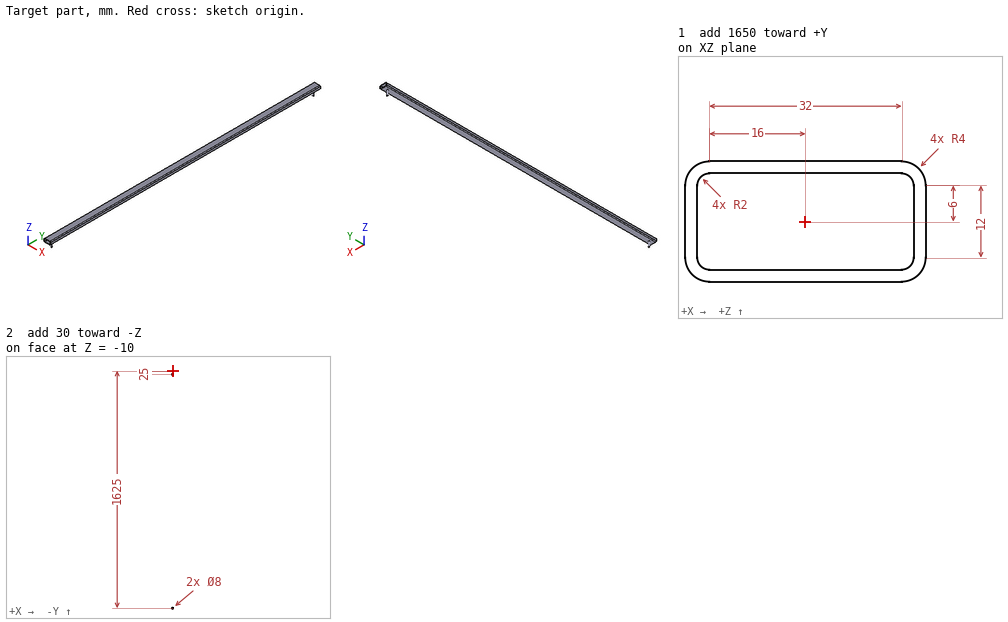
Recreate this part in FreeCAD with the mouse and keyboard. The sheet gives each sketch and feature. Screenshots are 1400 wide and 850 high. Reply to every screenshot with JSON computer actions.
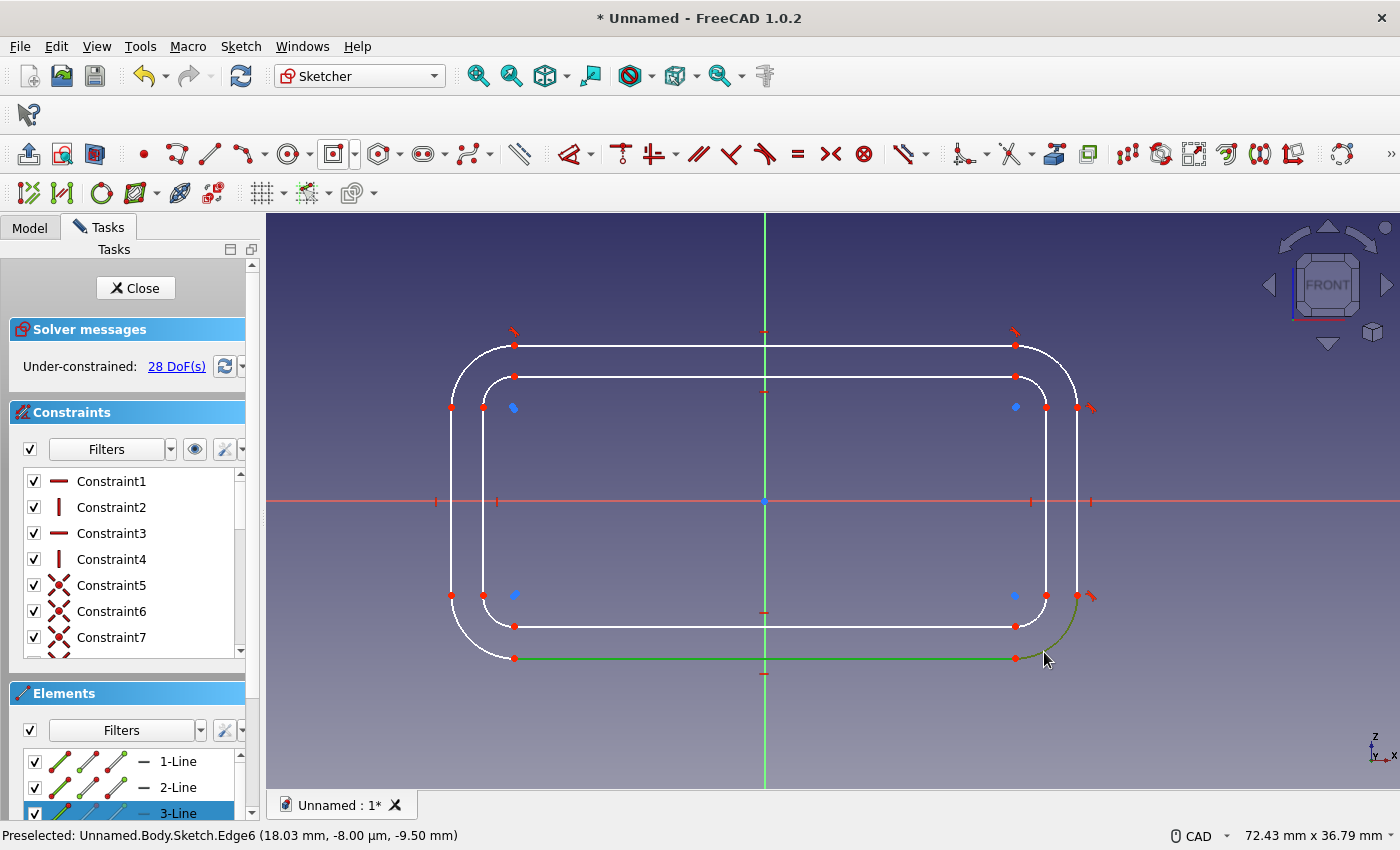
{"action": "left_click", "coordinate": [765, 154]}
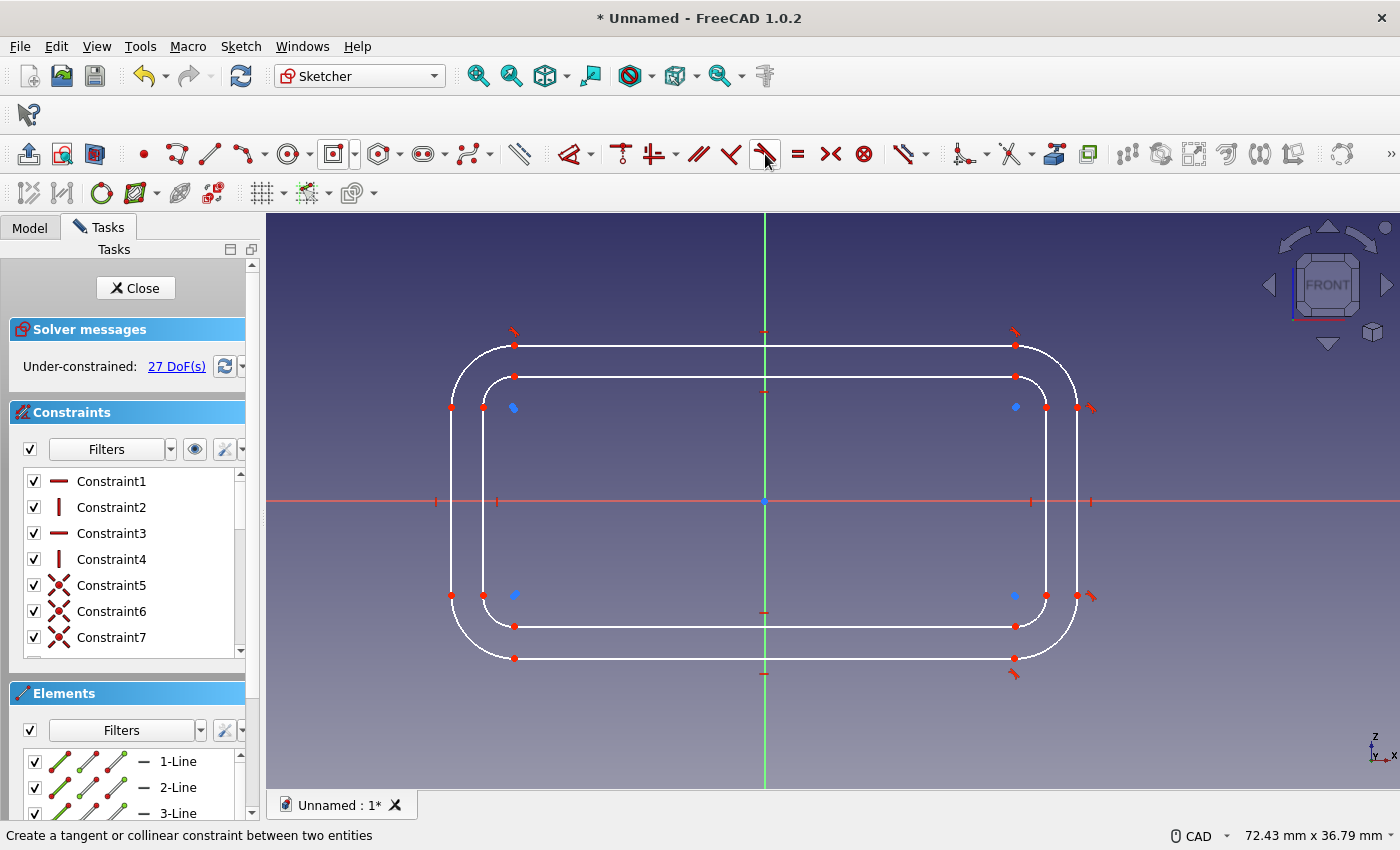
{"action": "left_click", "coordinate": [864, 659]}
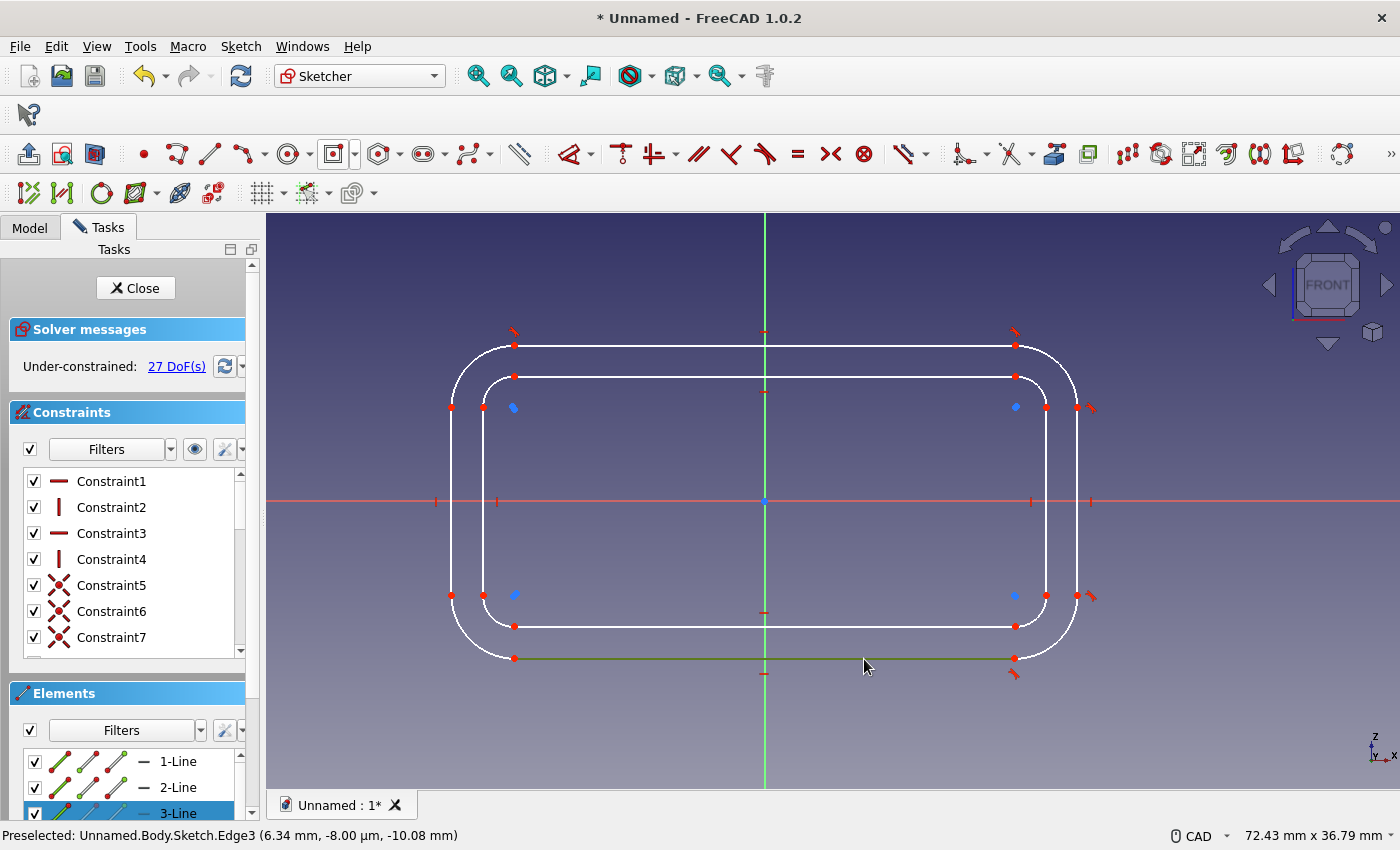
{"action": "left_click", "coordinate": [459, 624]}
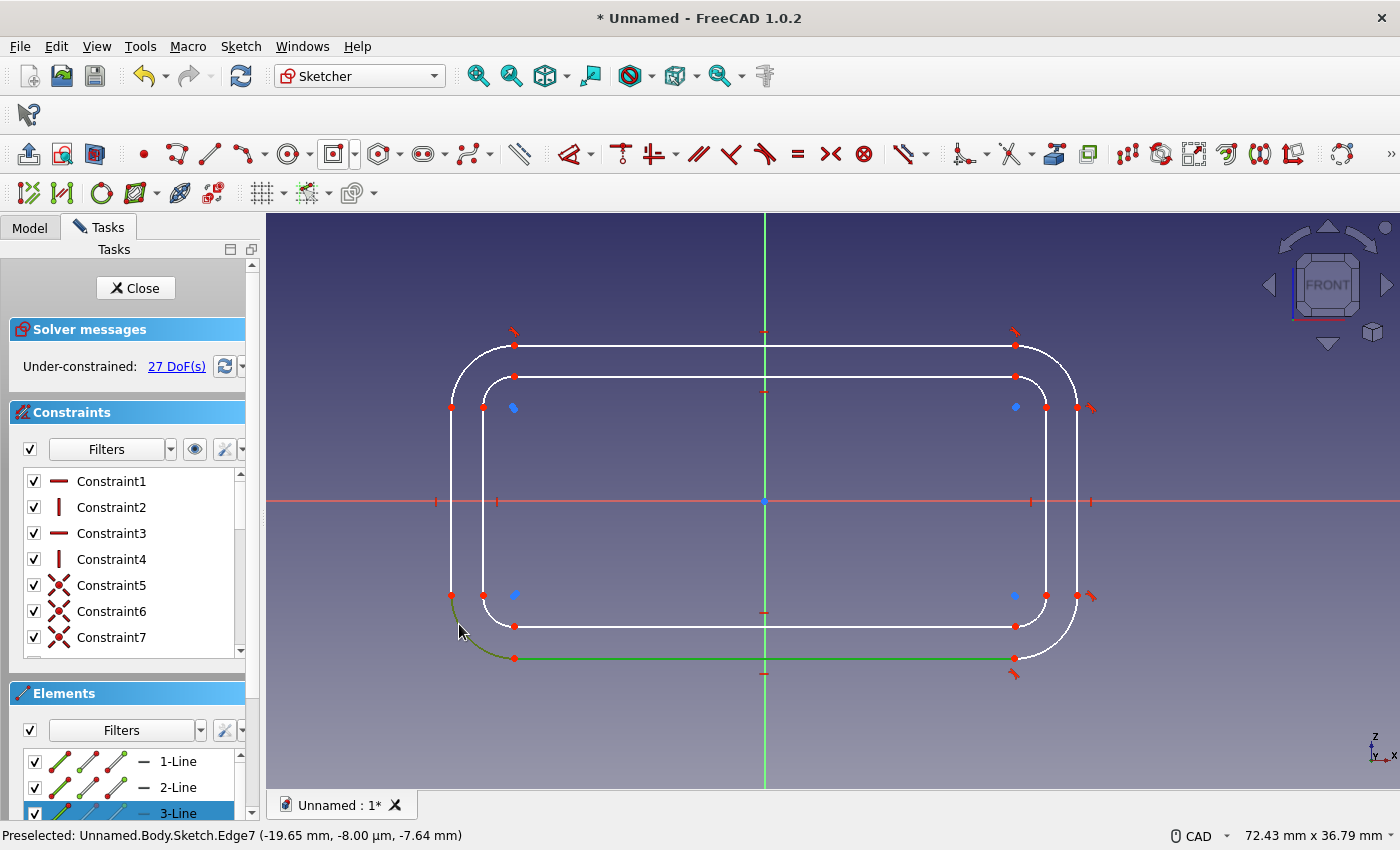
{"action": "left_click", "coordinate": [765, 154]}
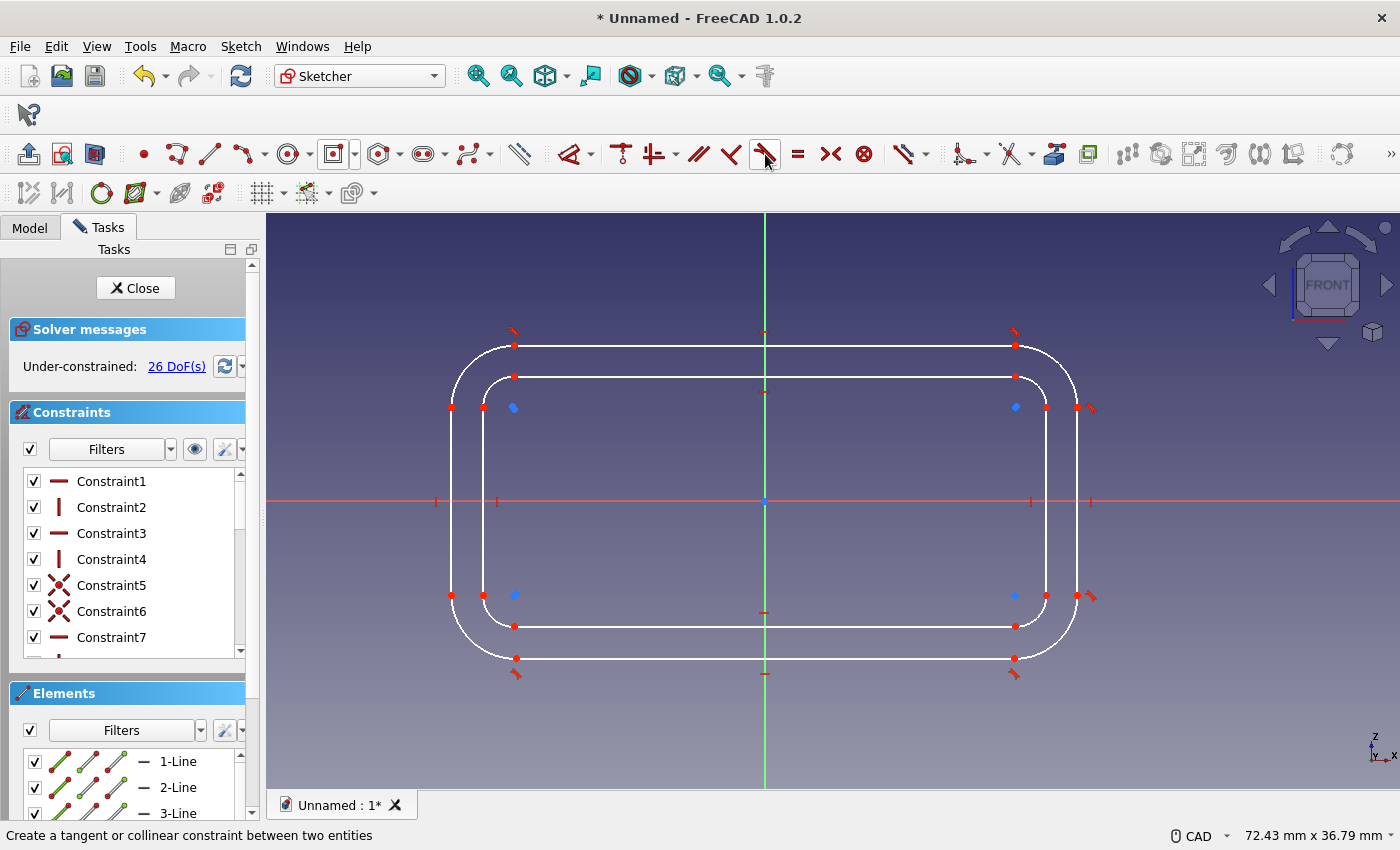
{"action": "left_click", "coordinate": [451, 540]}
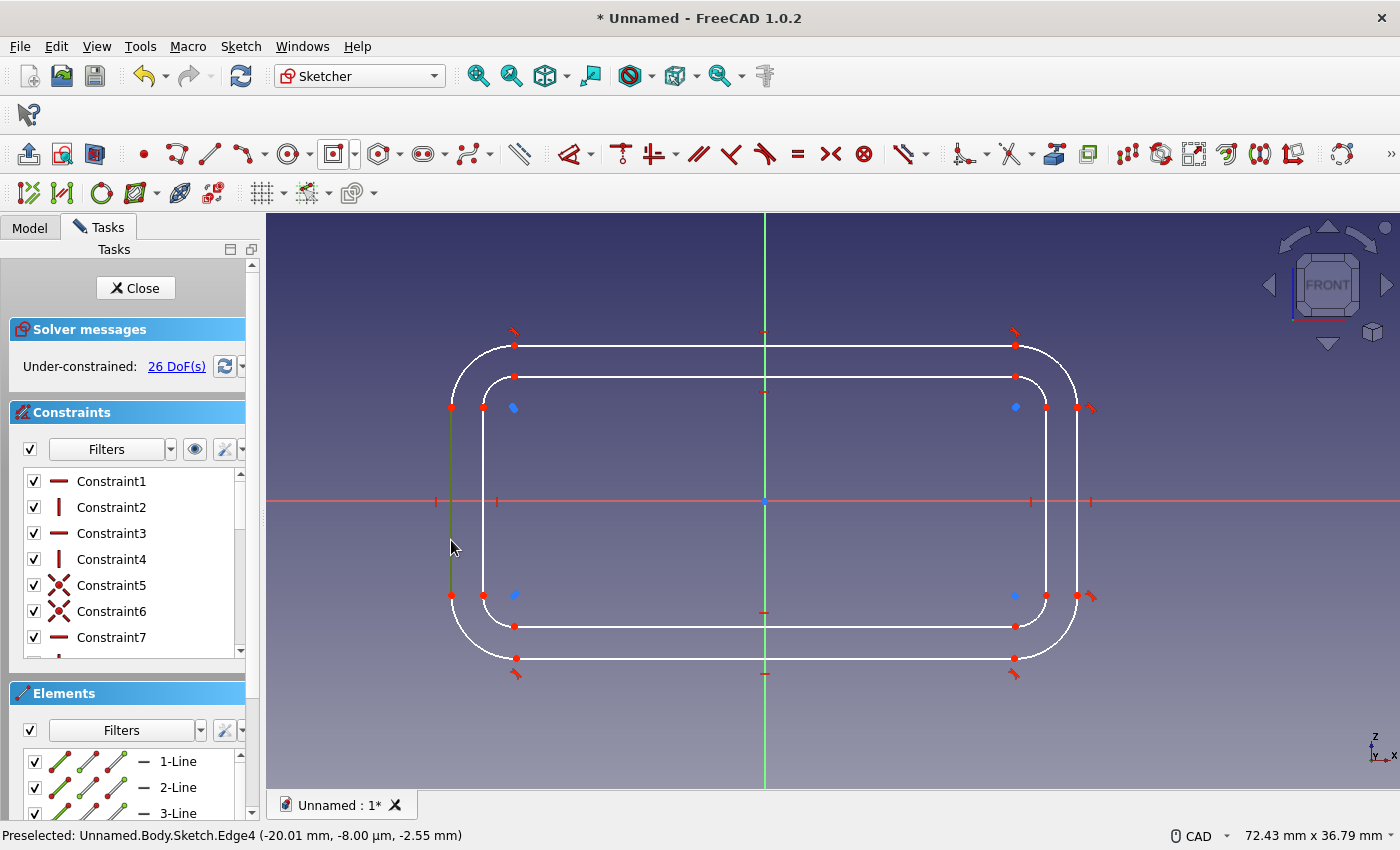
{"action": "left_click", "coordinate": [459, 625]}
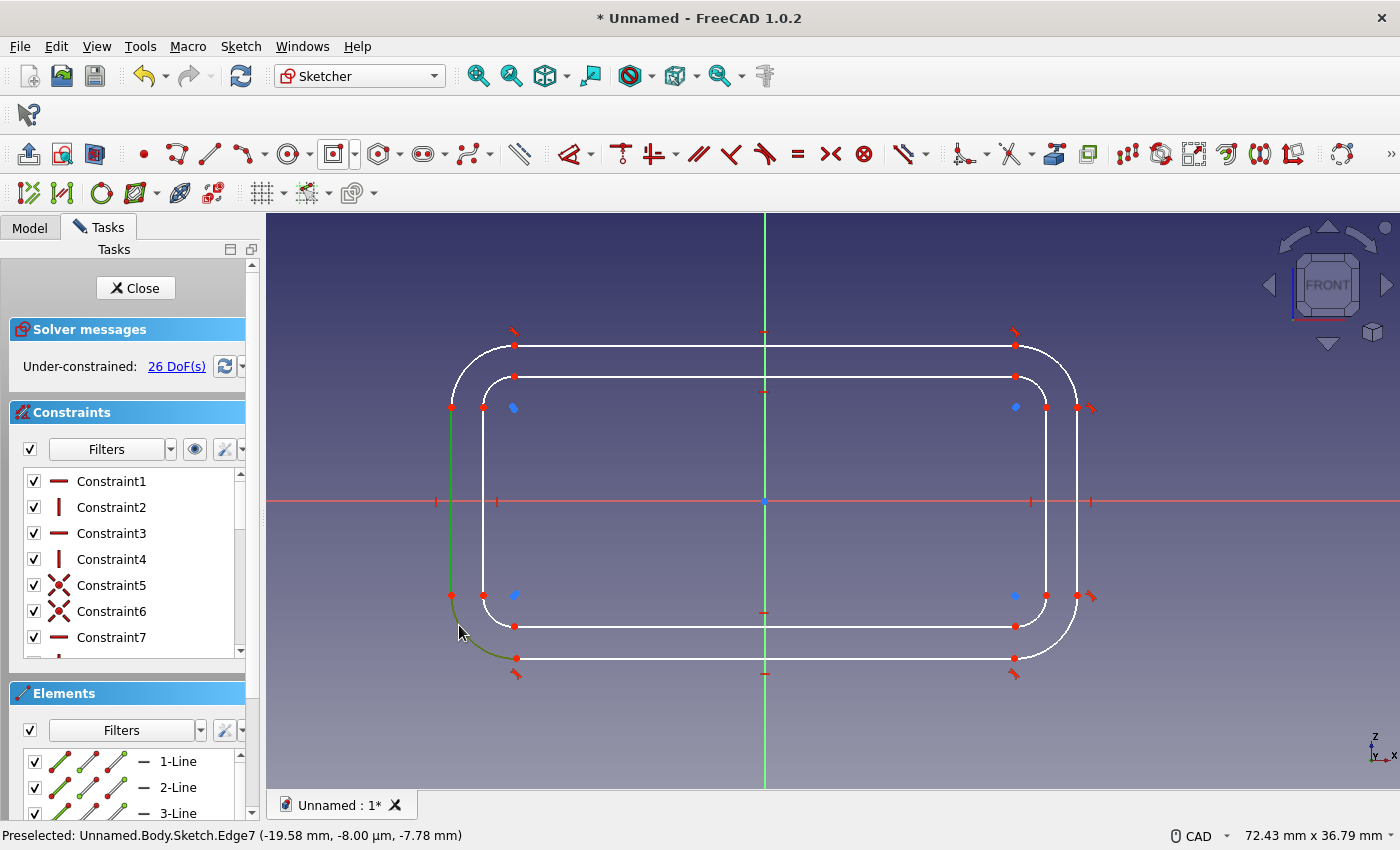
{"action": "left_click", "coordinate": [765, 154]}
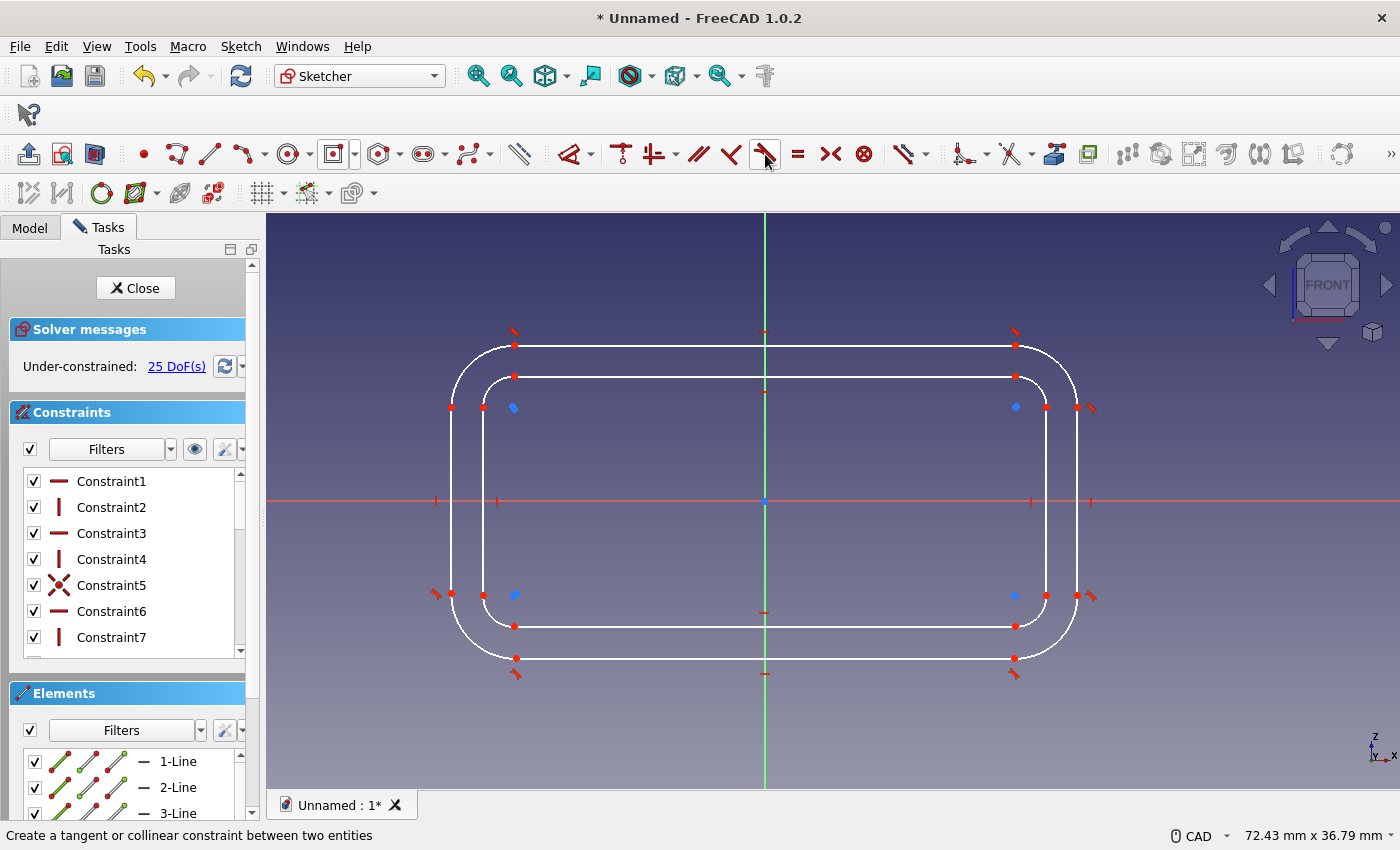
{"action": "left_click", "coordinate": [451, 538]}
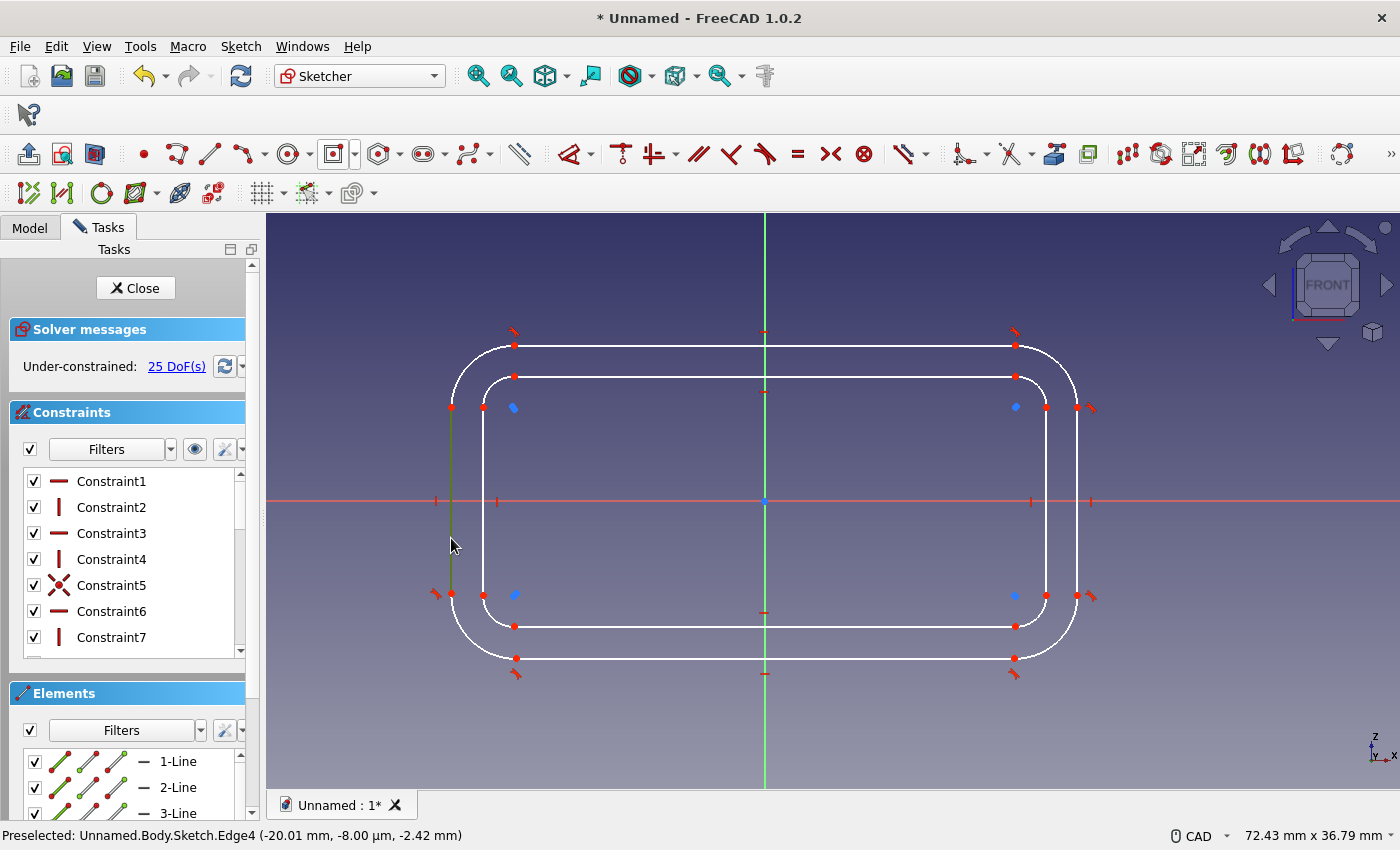
{"action": "left_click", "coordinate": [486, 353]}